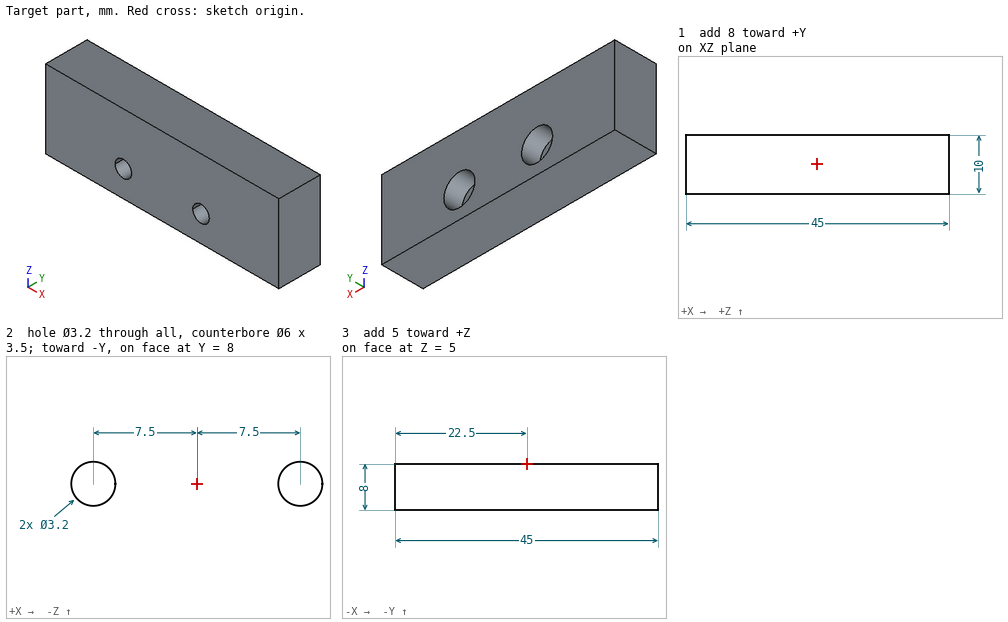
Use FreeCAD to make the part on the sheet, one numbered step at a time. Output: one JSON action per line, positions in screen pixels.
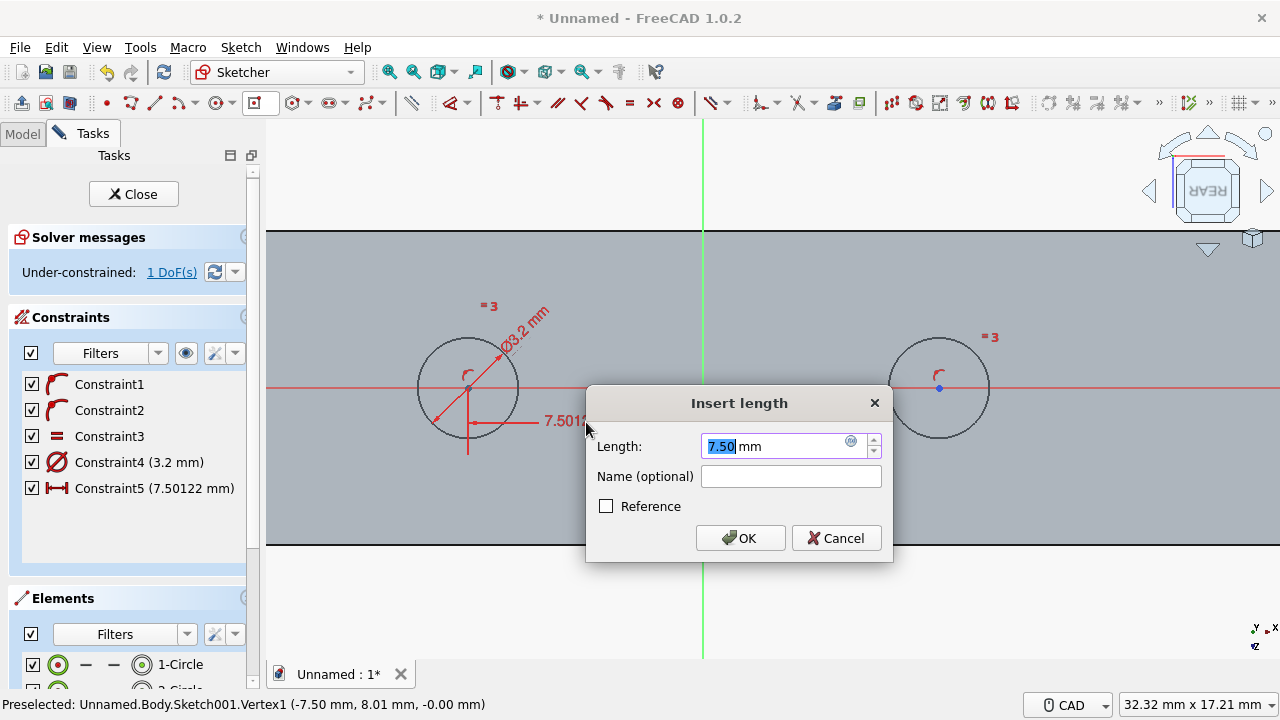
{"action": "type", "text": "7.5"}
{"action": "key", "text": "Return"}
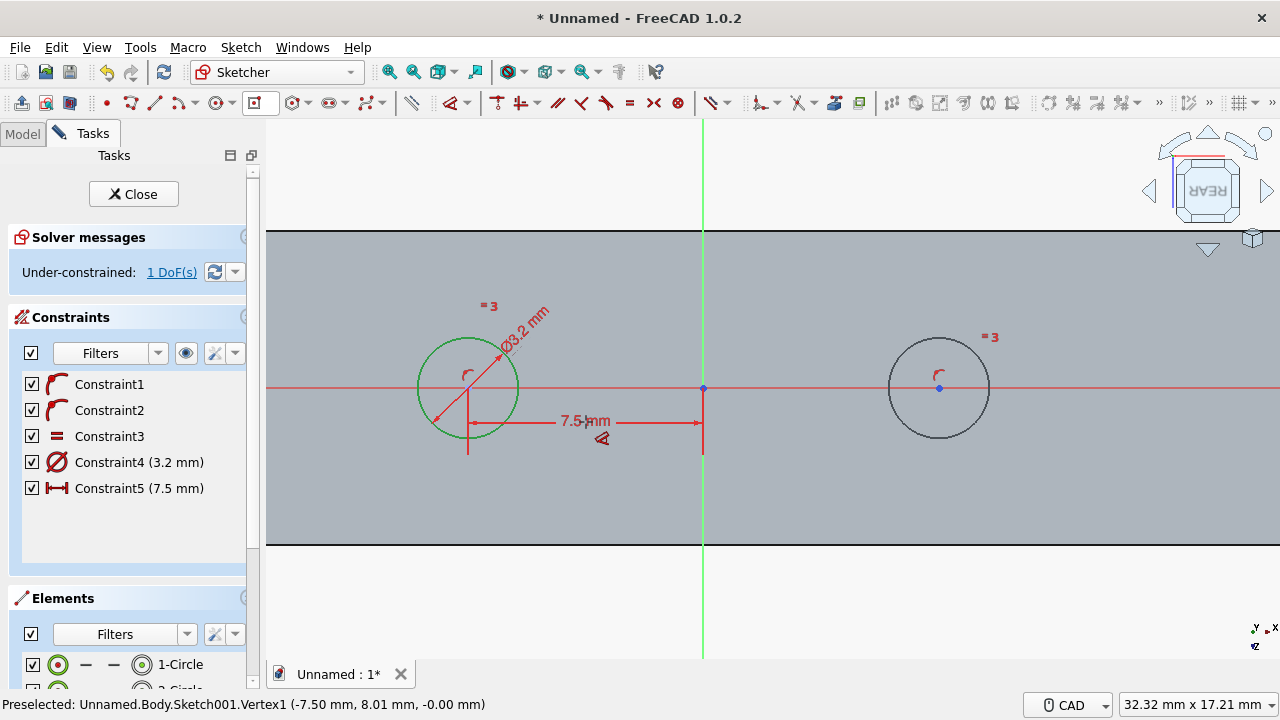
{"action": "left_click", "coordinate": [939, 388]}
{"action": "left_click", "coordinate": [821, 422]}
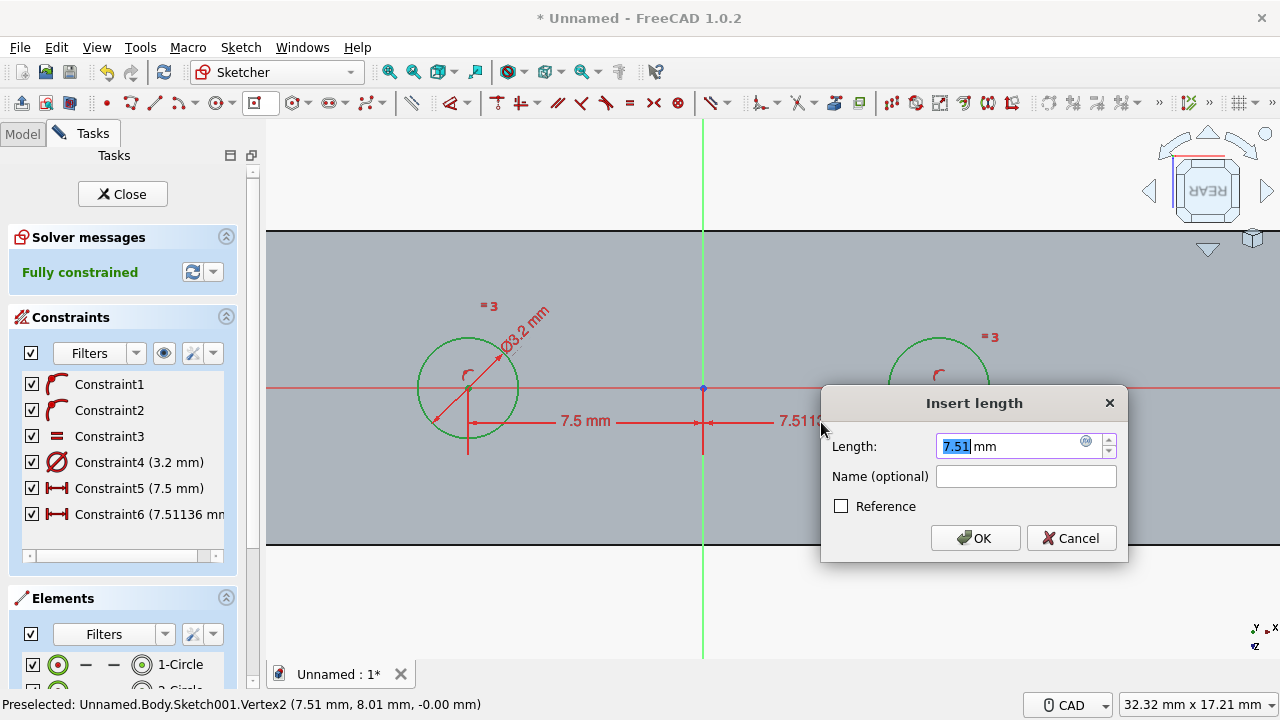
{"action": "type", "text": "7.5"}
{"action": "key", "text": "Return"}
{"action": "key", "text": "Escape"}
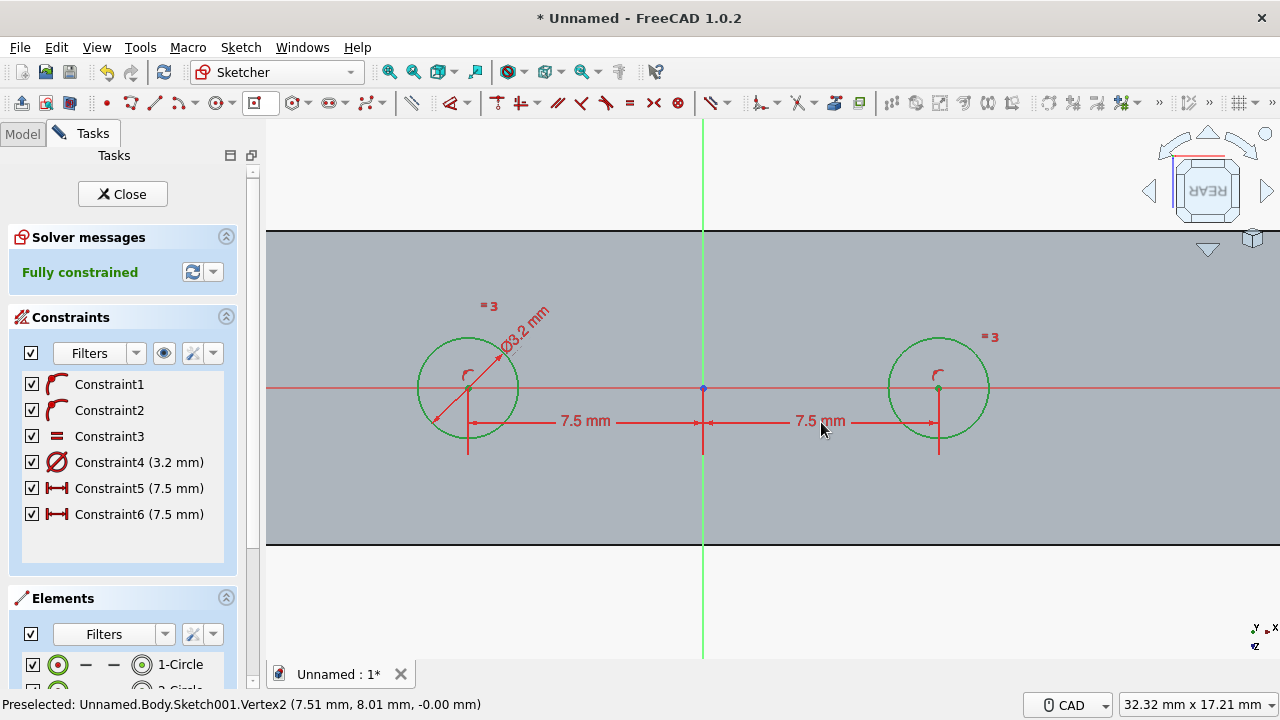
{"action": "left_click", "coordinate": [123, 194]}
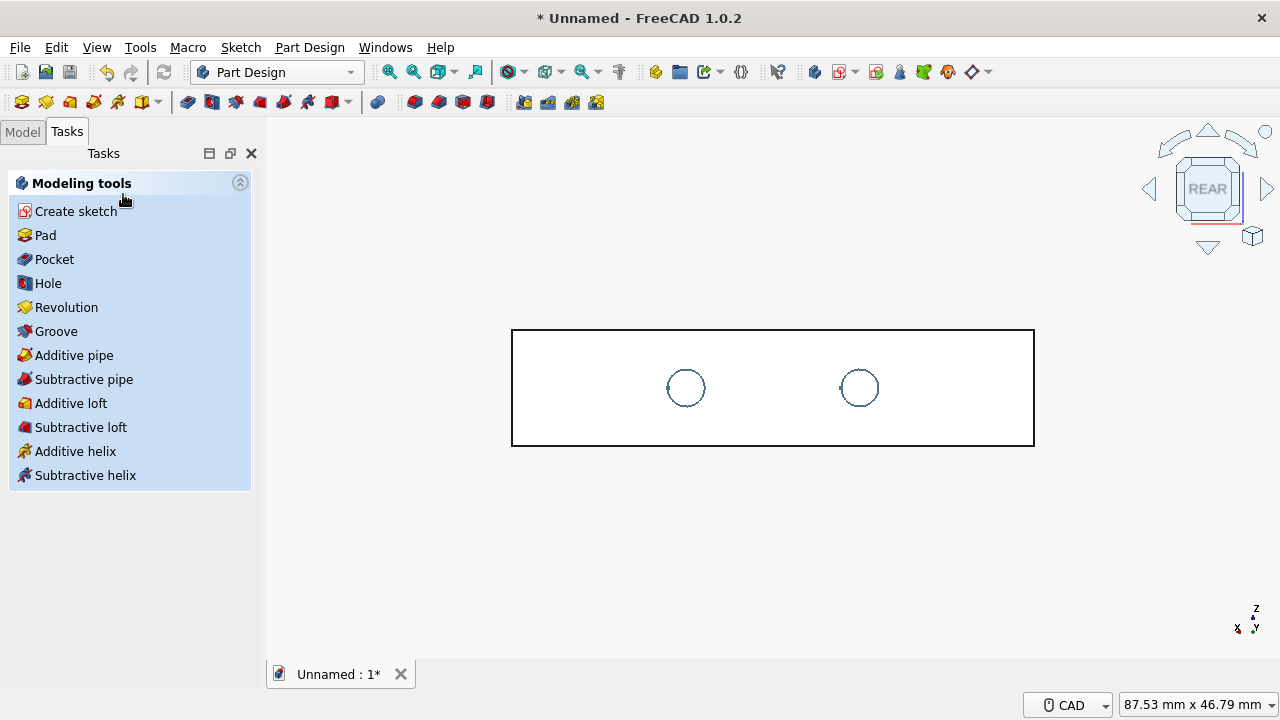
{"action": "left_click", "coordinate": [212, 102]}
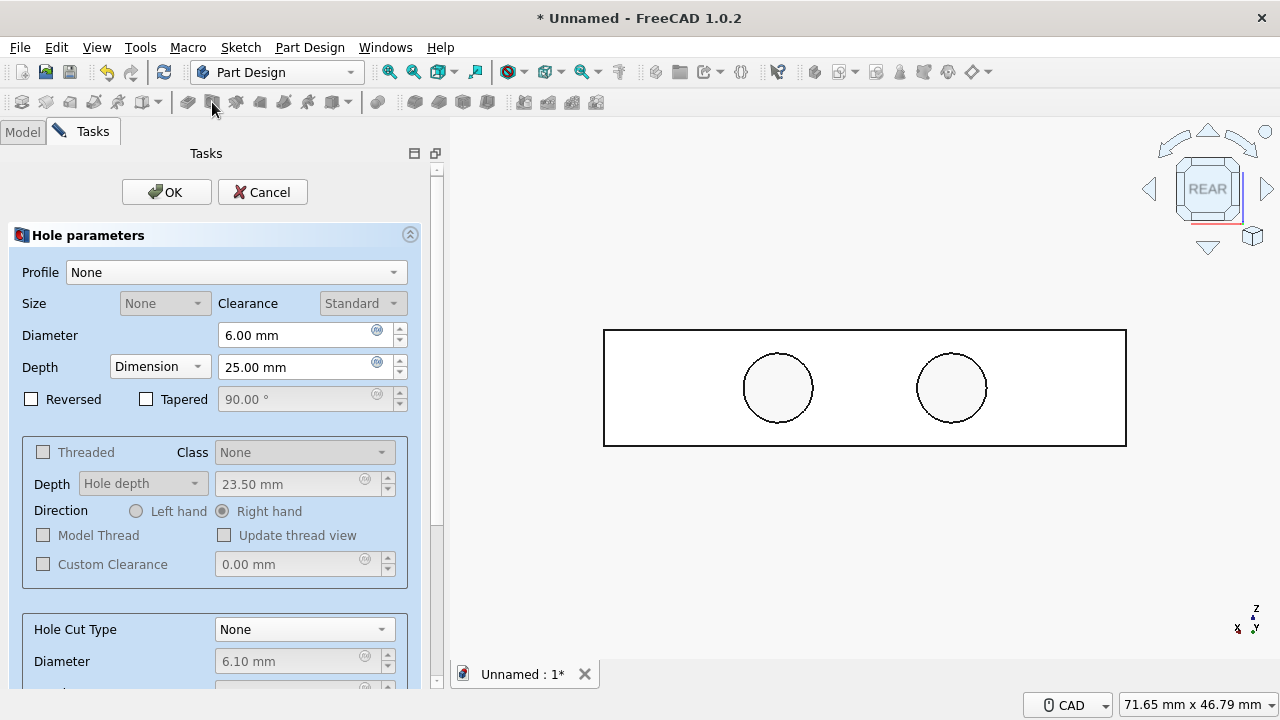
{"action": "triple_click", "coordinate": [305, 335]}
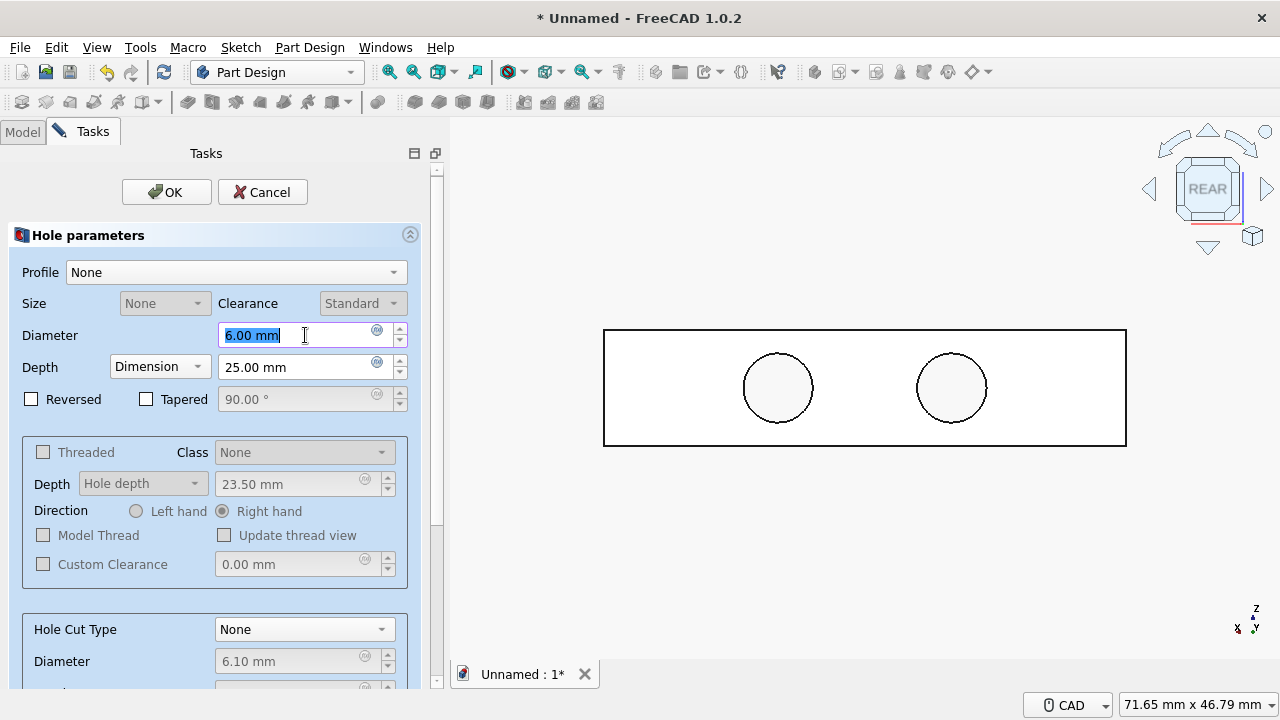
{"action": "type", "text": "3.2"}
{"action": "key", "text": "Tab"}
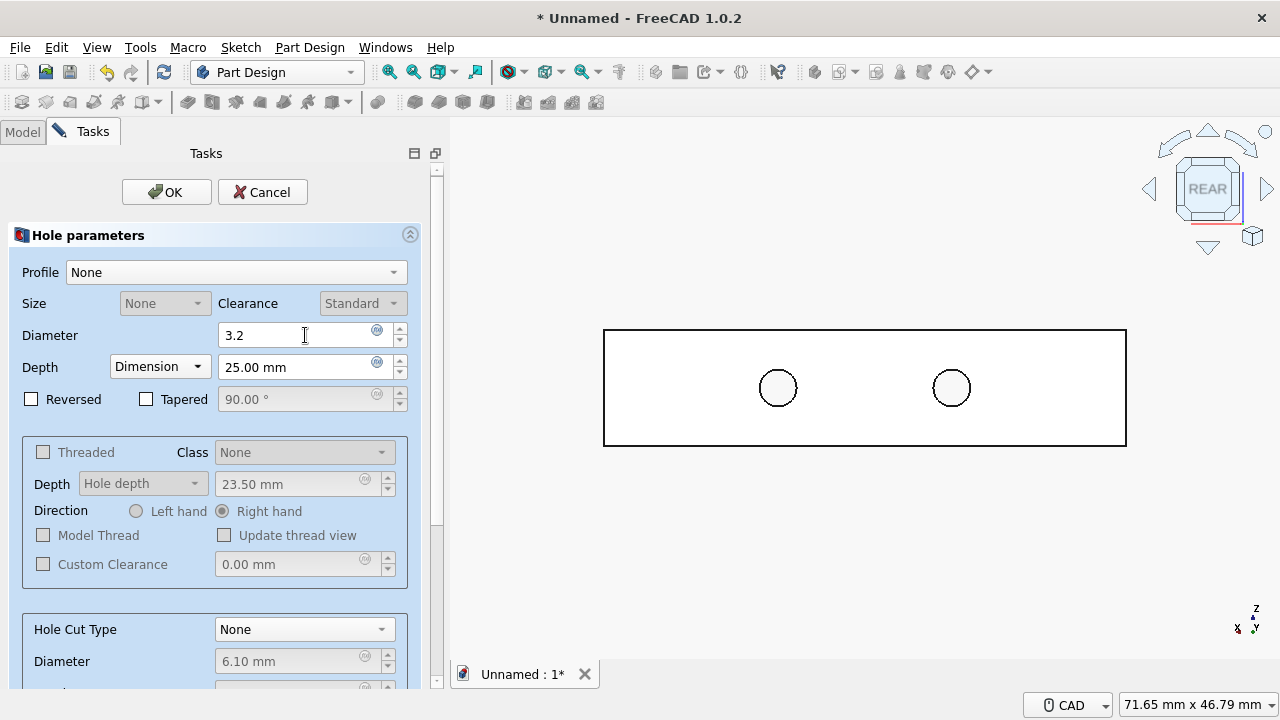
{"action": "left_click", "coordinate": [161, 366]}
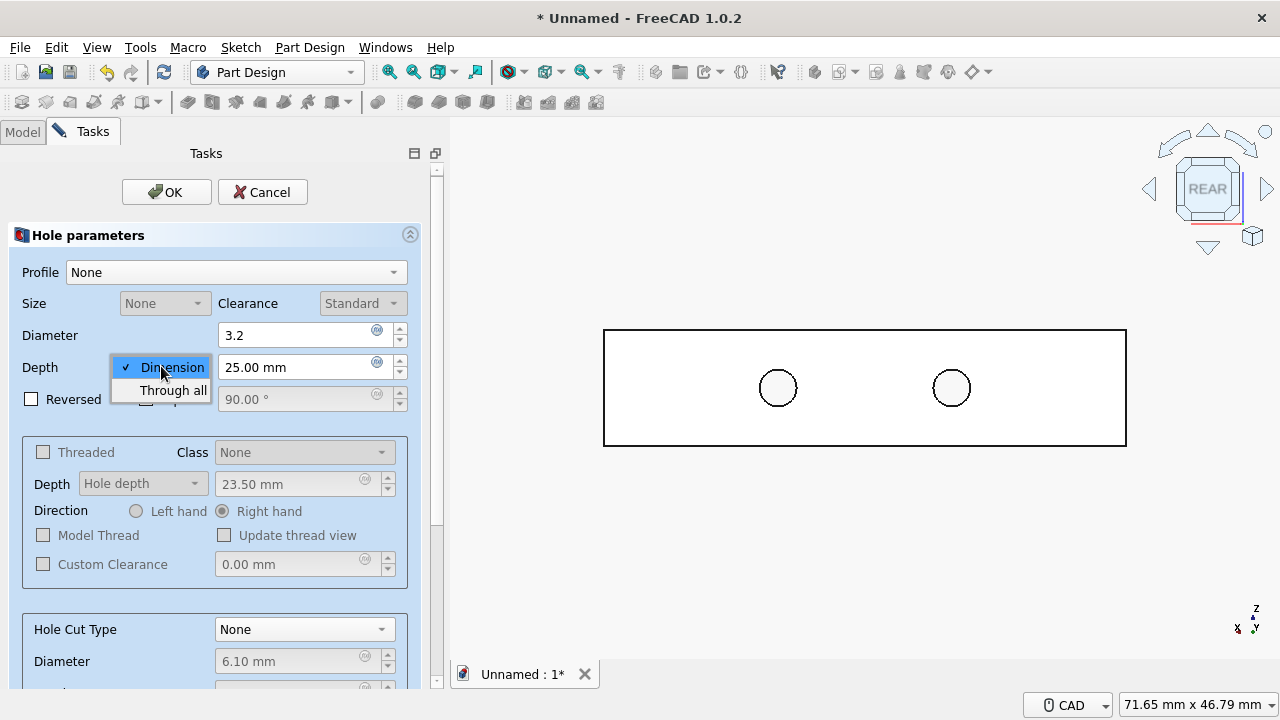
{"action": "left_click", "coordinate": [160, 390]}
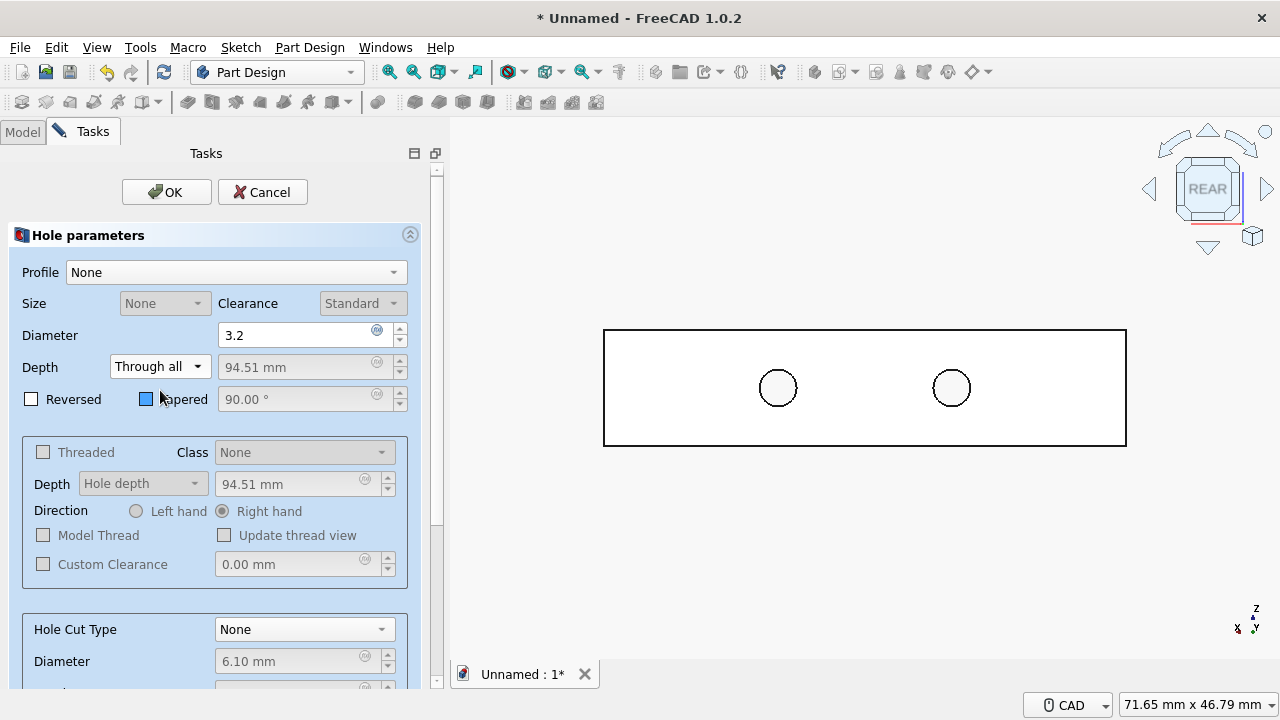
{"action": "left_click", "coordinate": [306, 630]}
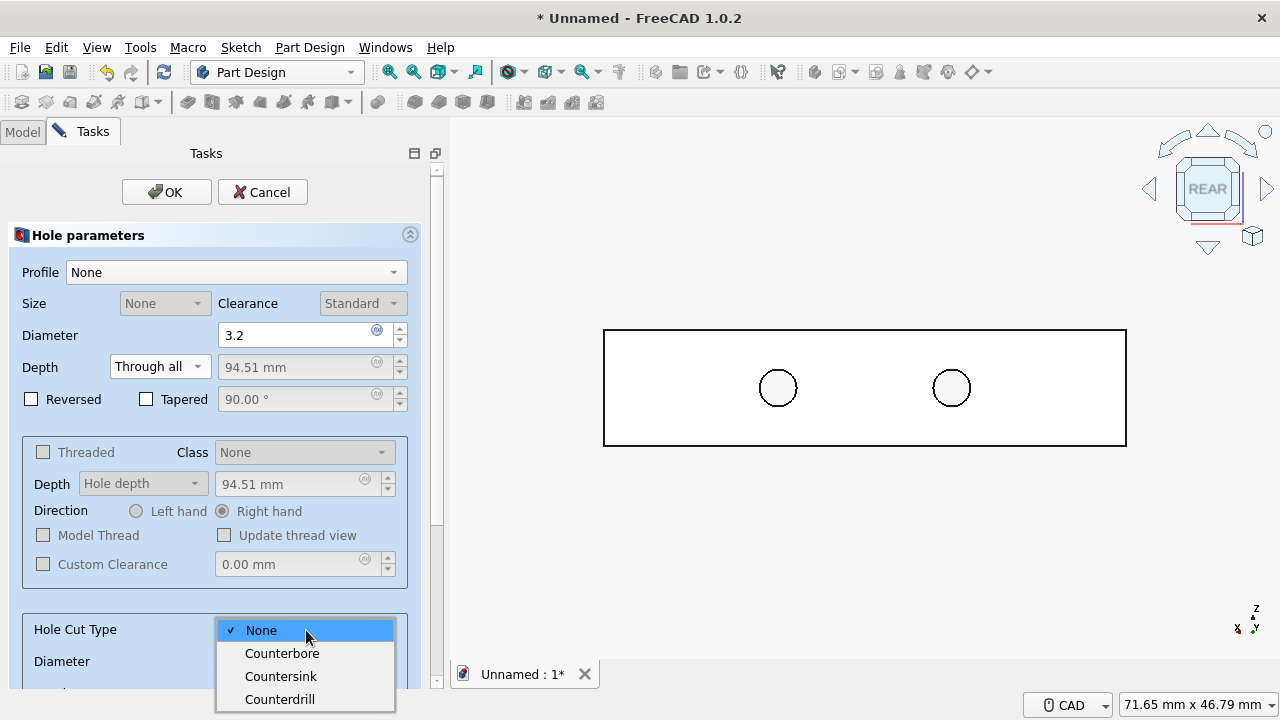
{"action": "left_click", "coordinate": [304, 654]}